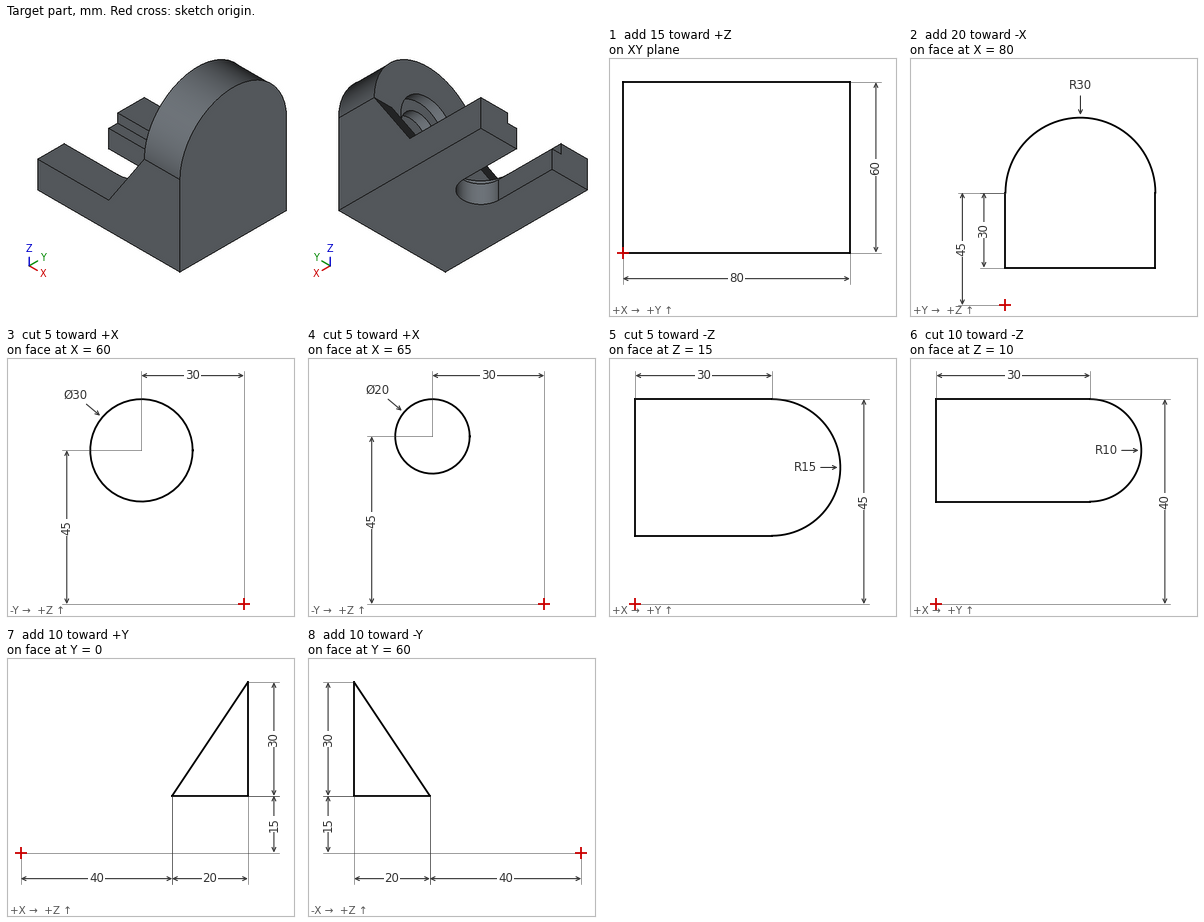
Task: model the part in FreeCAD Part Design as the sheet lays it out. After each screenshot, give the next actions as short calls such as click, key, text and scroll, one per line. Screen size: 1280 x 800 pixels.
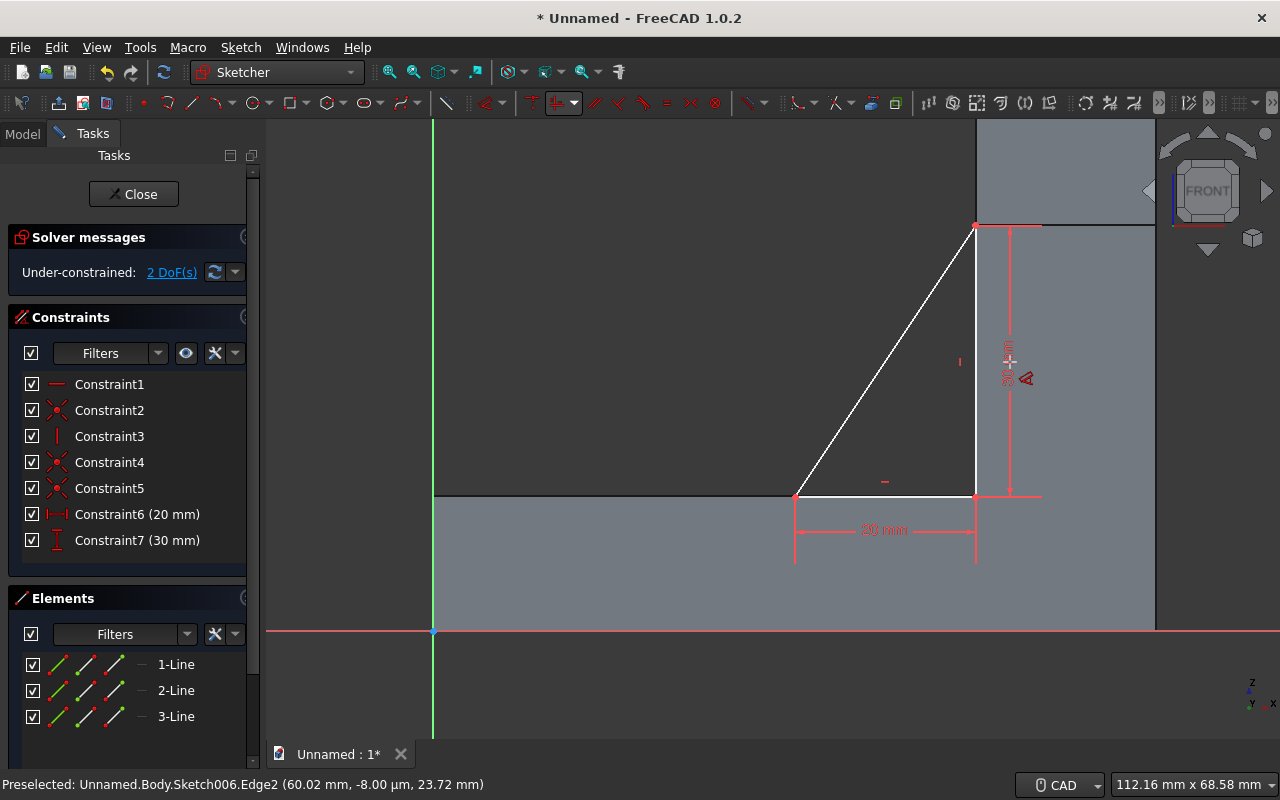
click(795, 497)
click(614, 665)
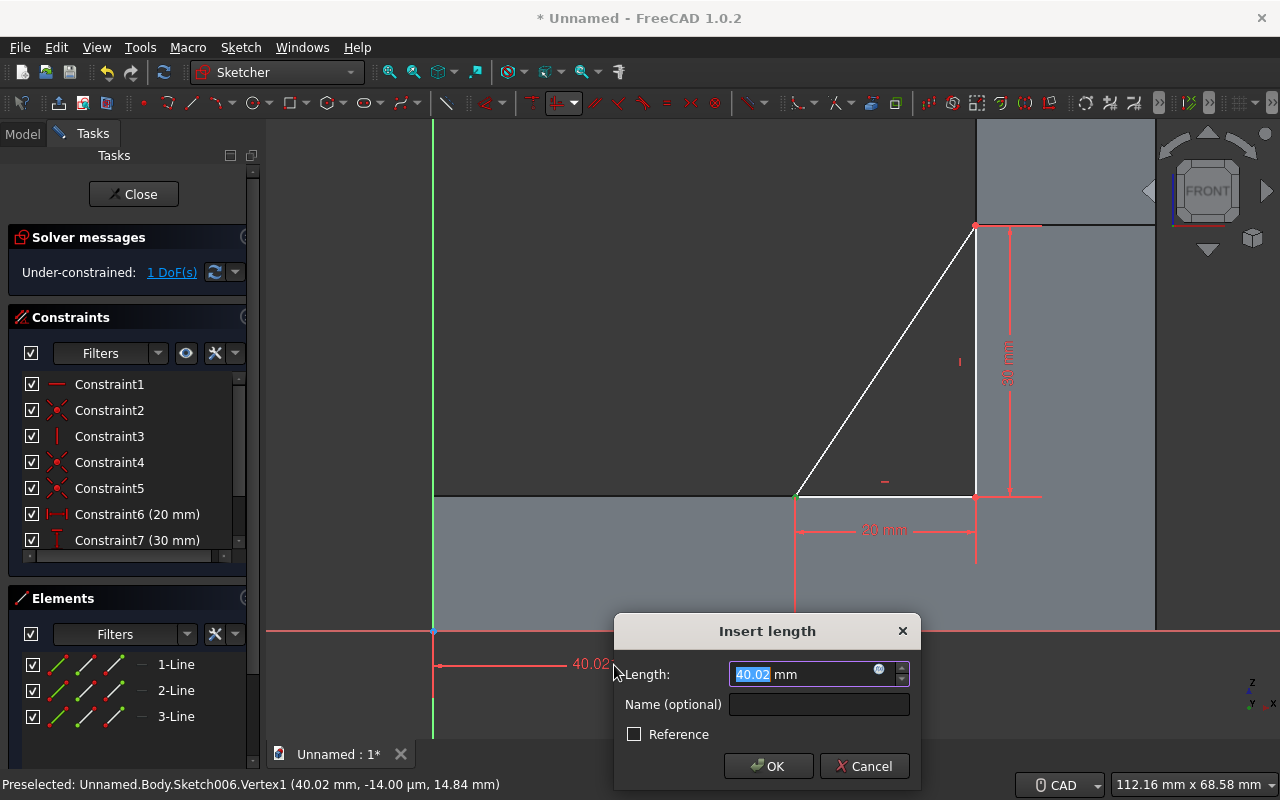
text(40)
key(Return)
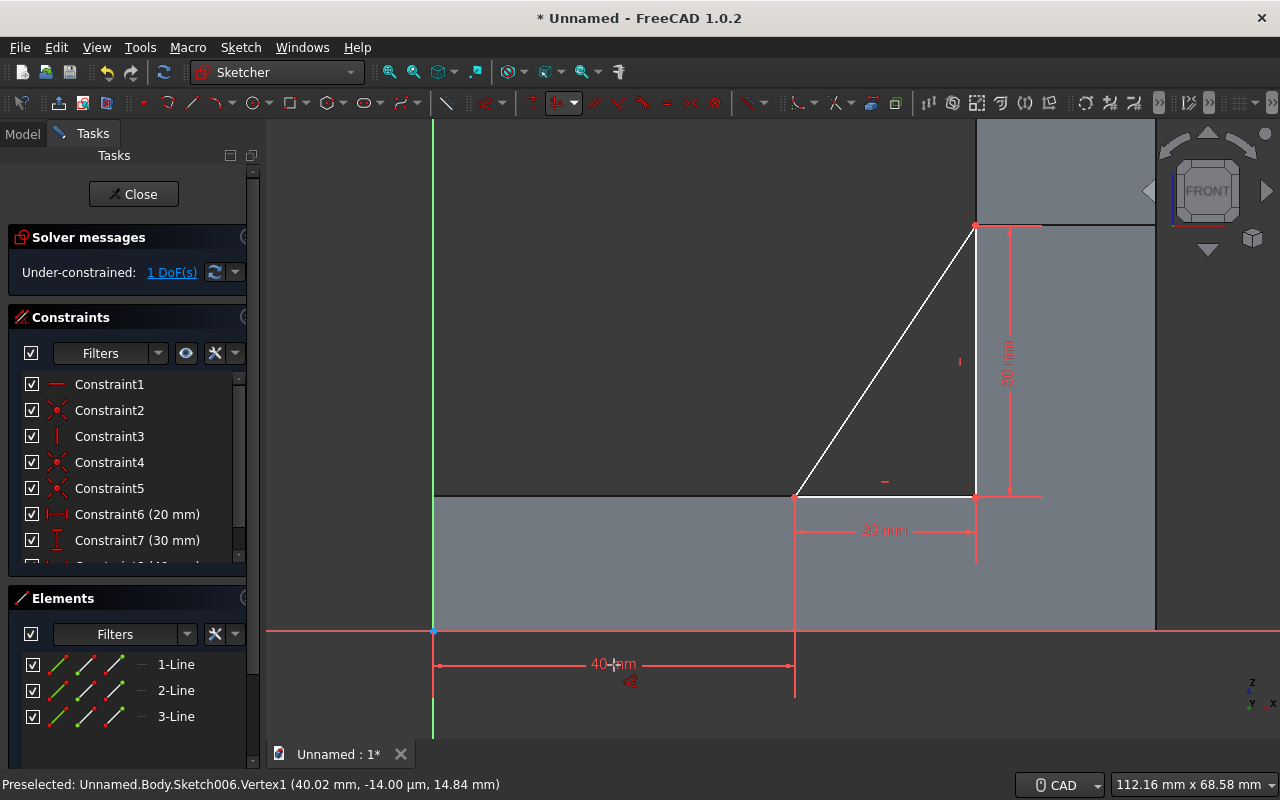
click(795, 497)
click(399, 564)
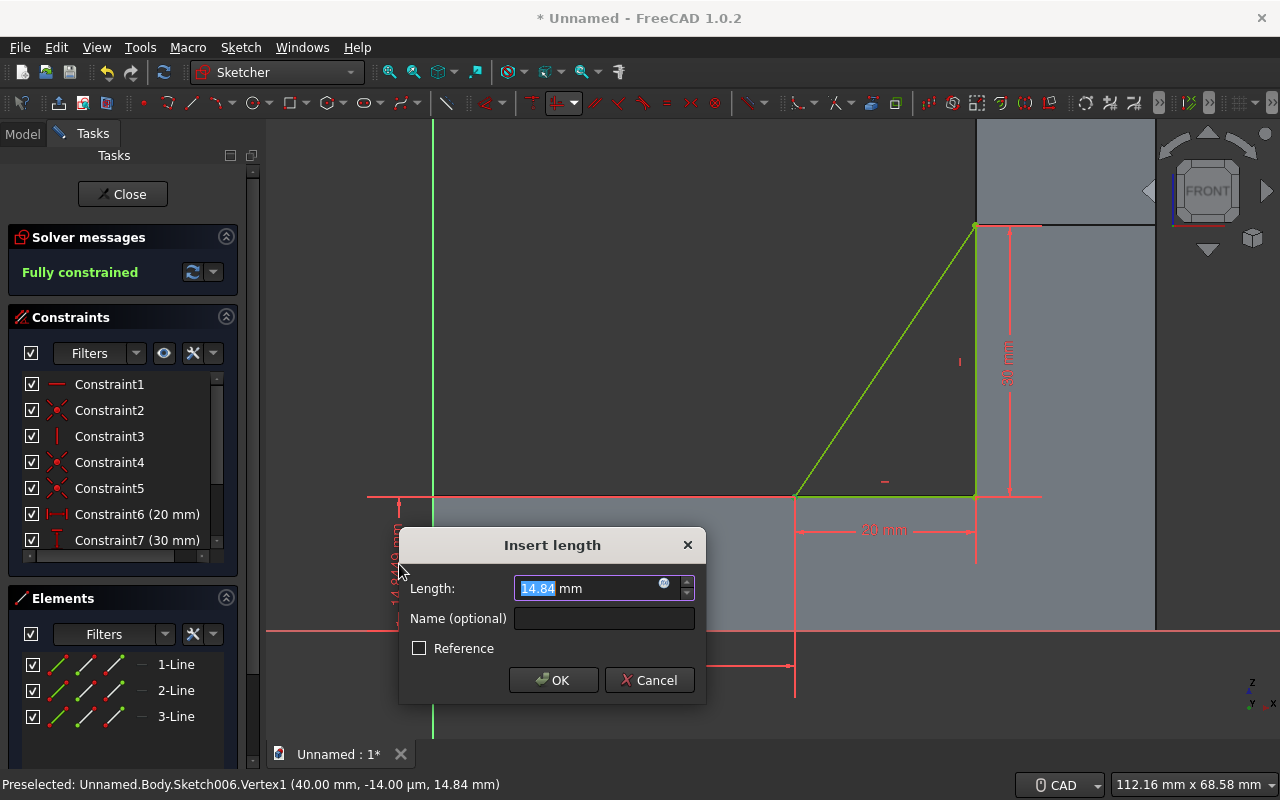
text(15)
key(Return)
key(Escape)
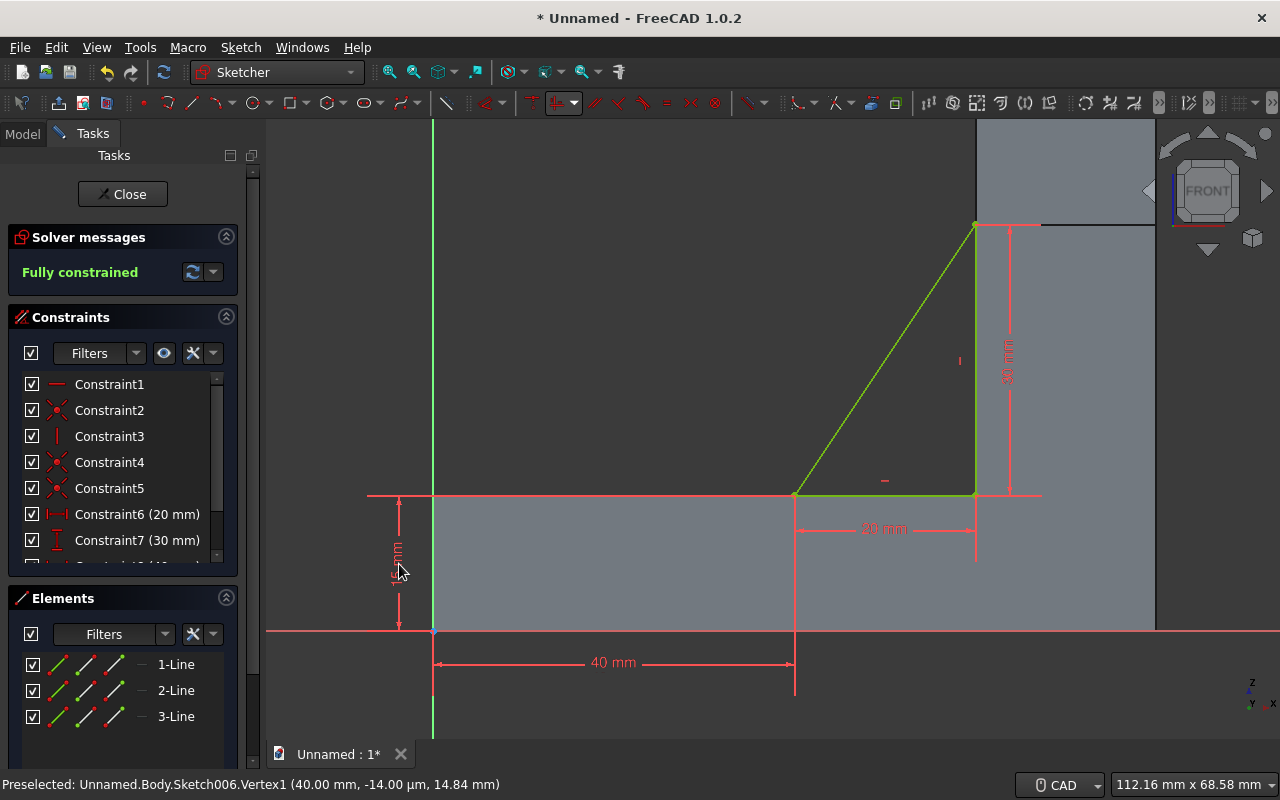
click(123, 194)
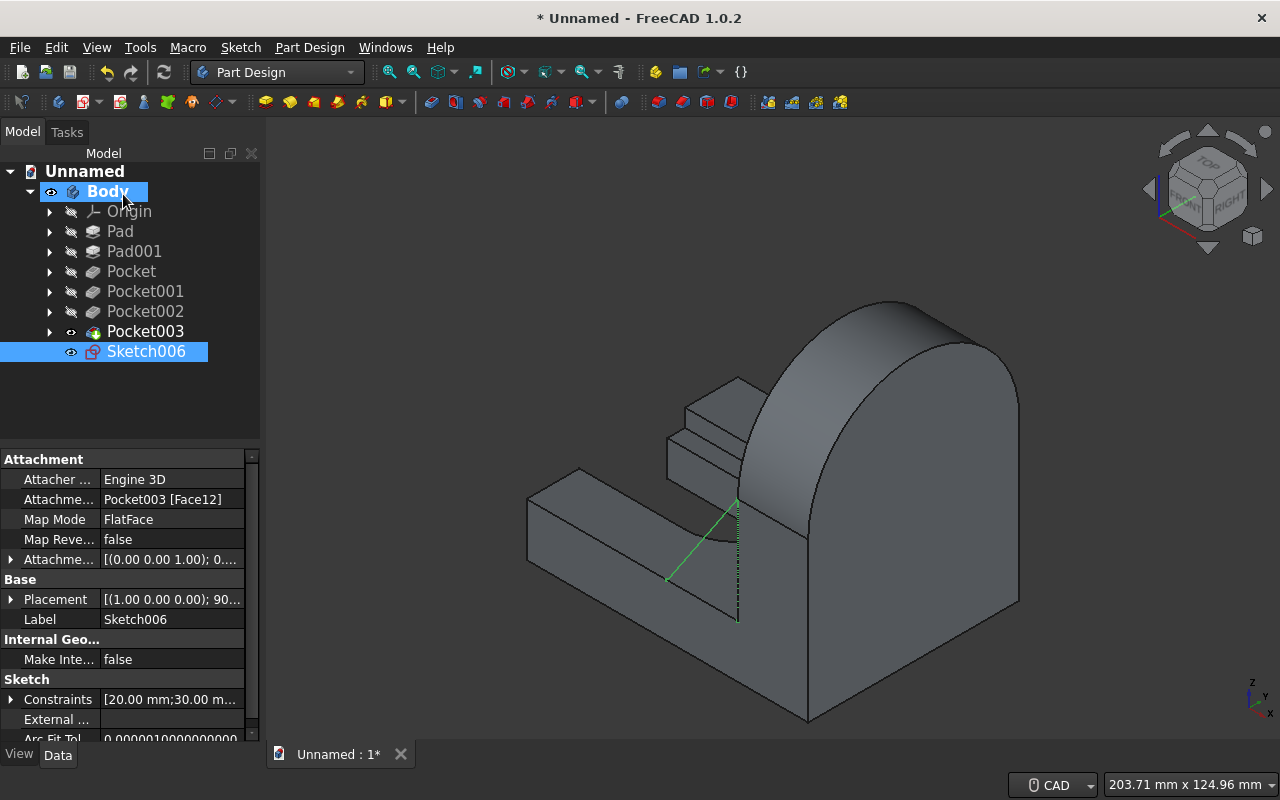
click(266, 102)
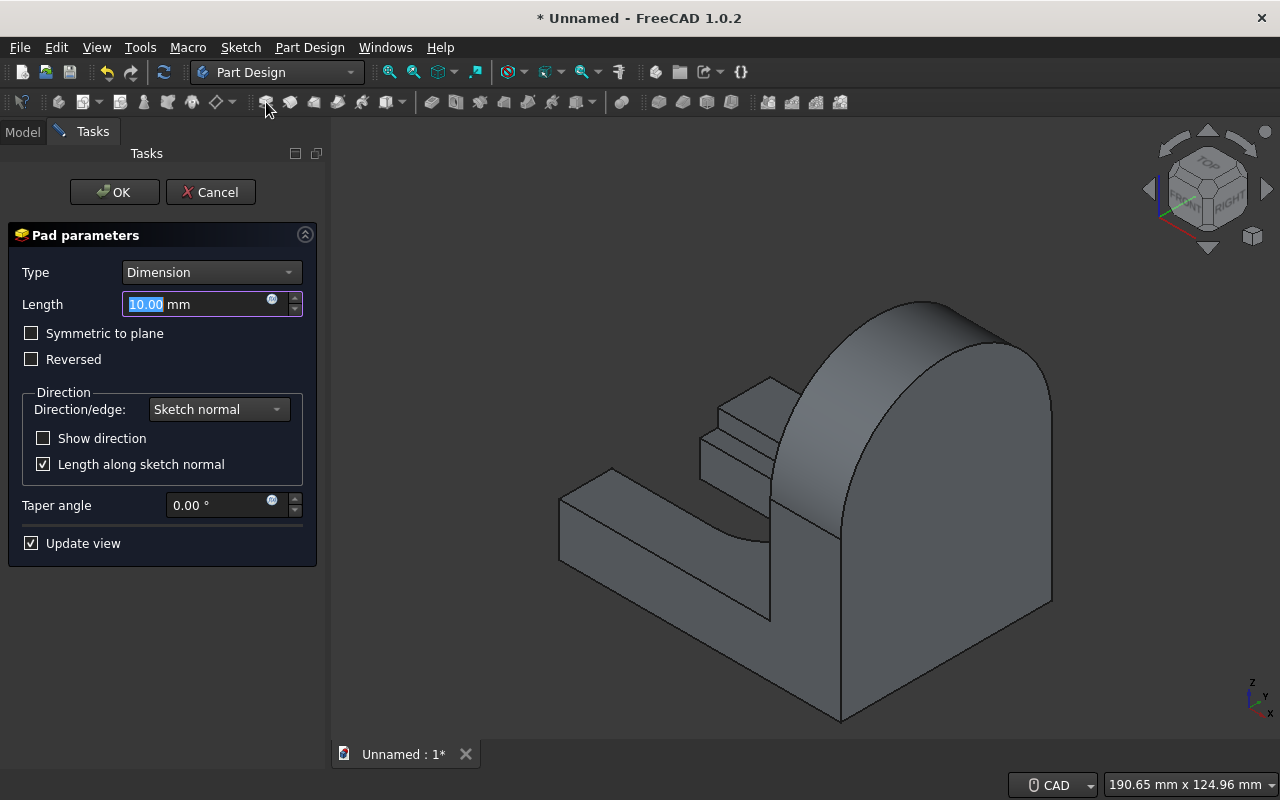
text(10)
key(Tab)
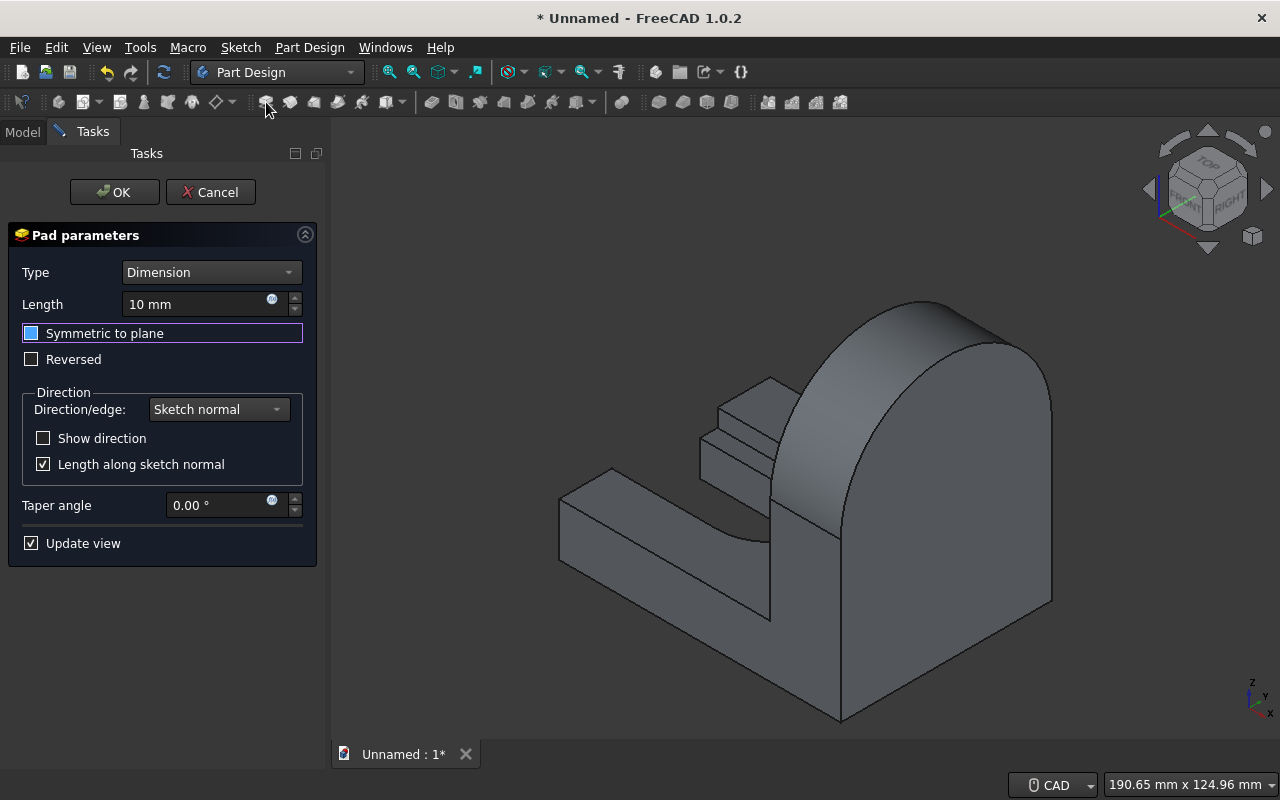
click(30, 359)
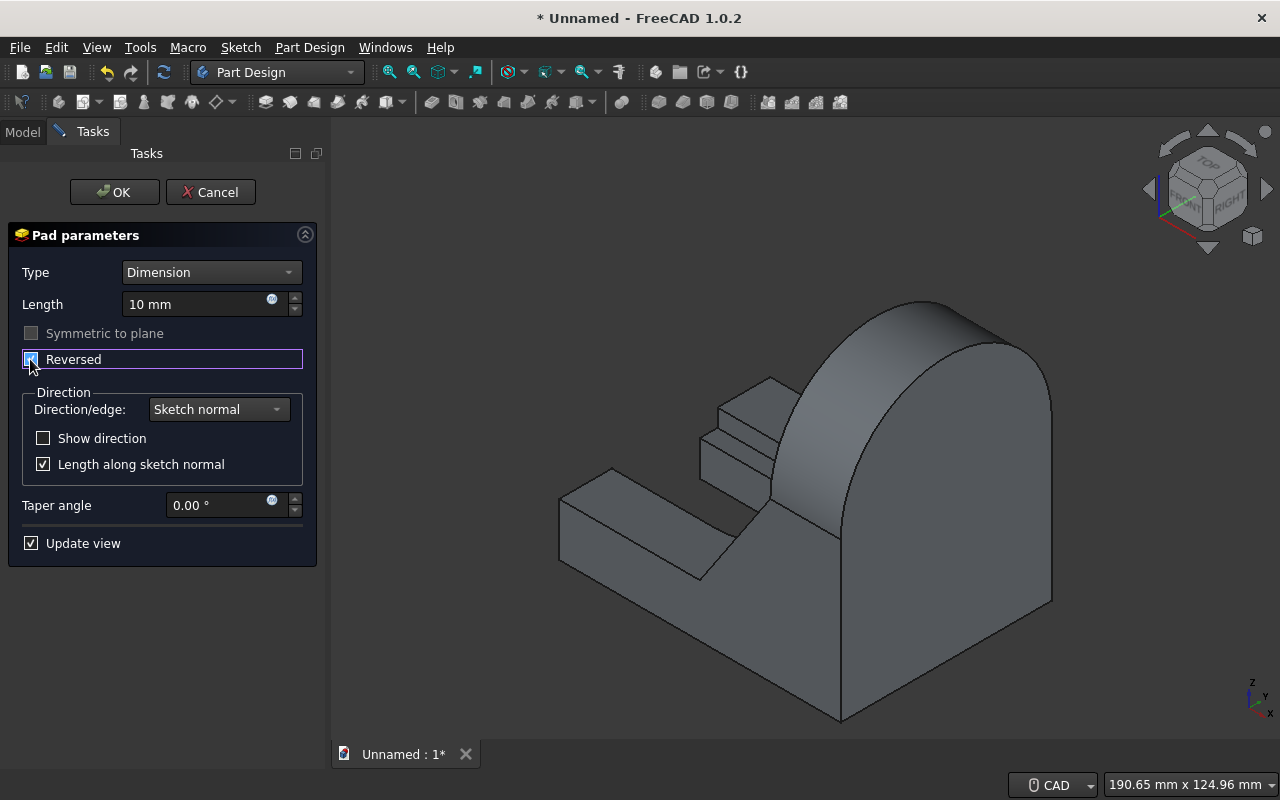
click(115, 192)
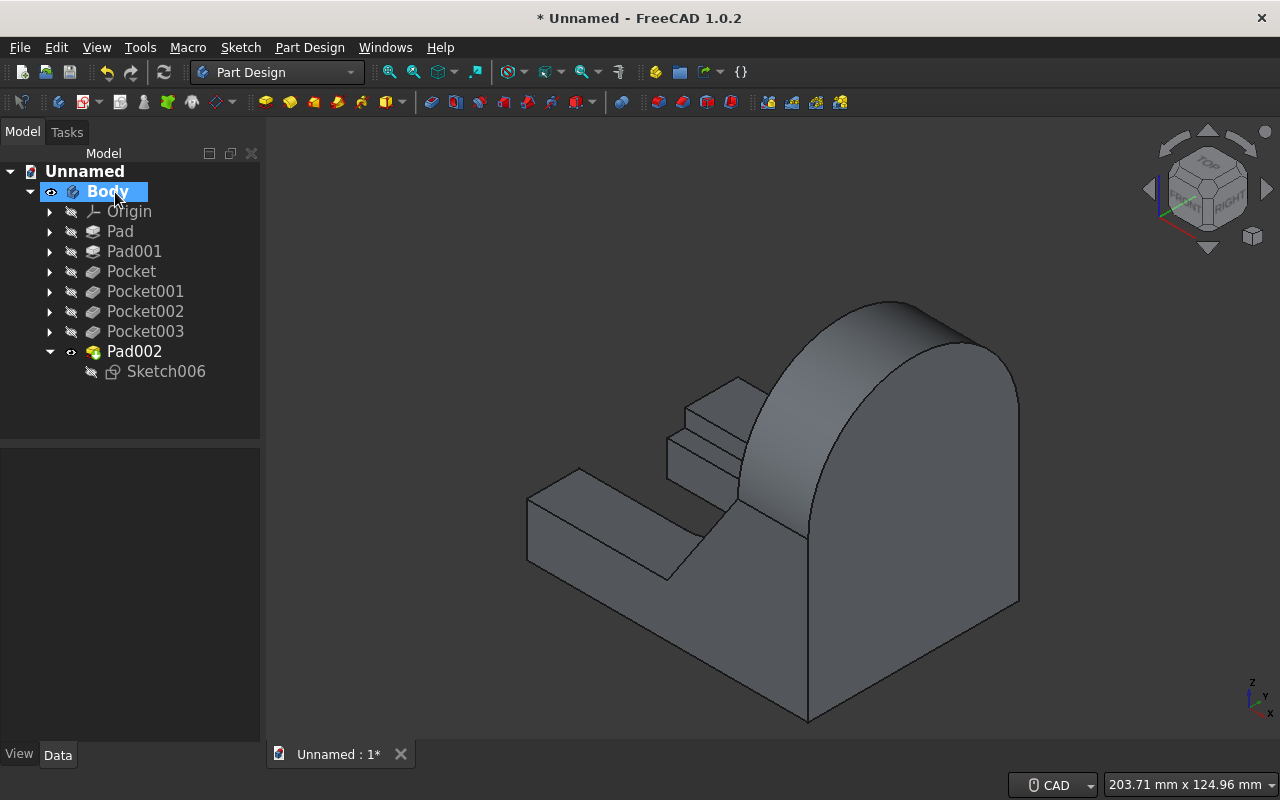
key(4)